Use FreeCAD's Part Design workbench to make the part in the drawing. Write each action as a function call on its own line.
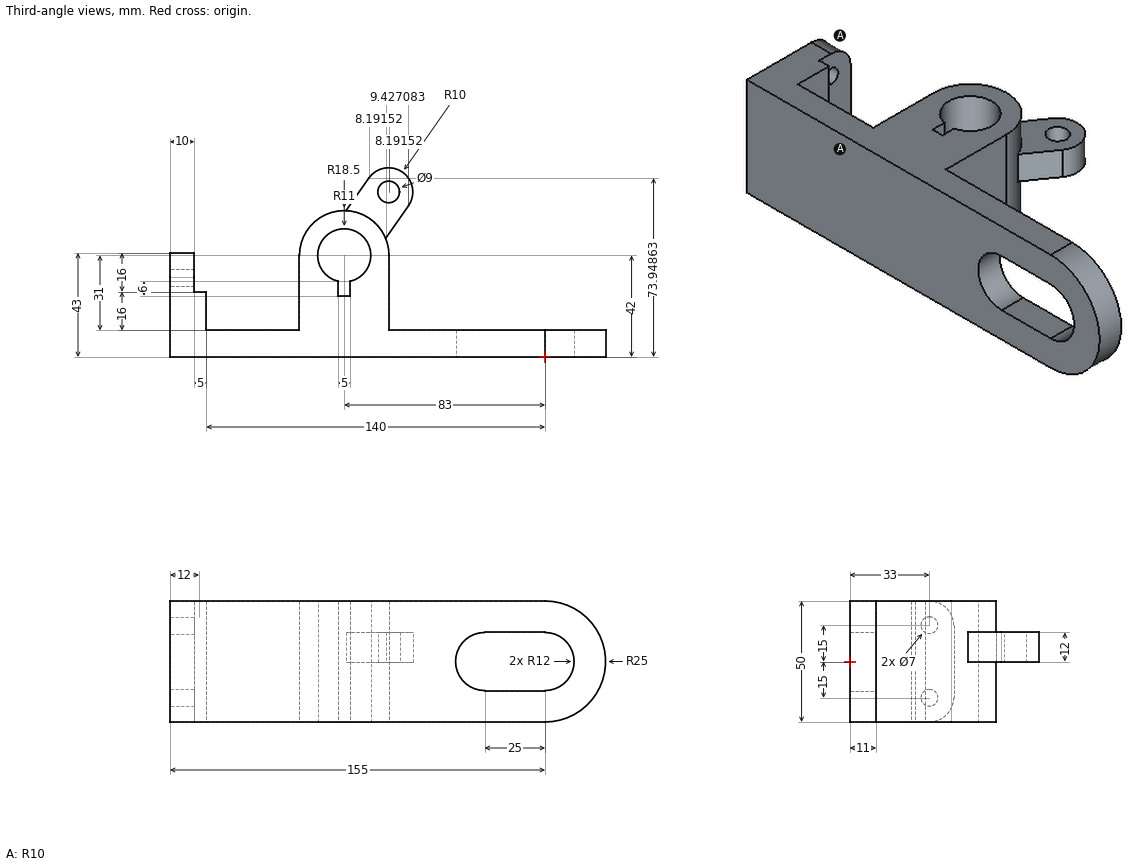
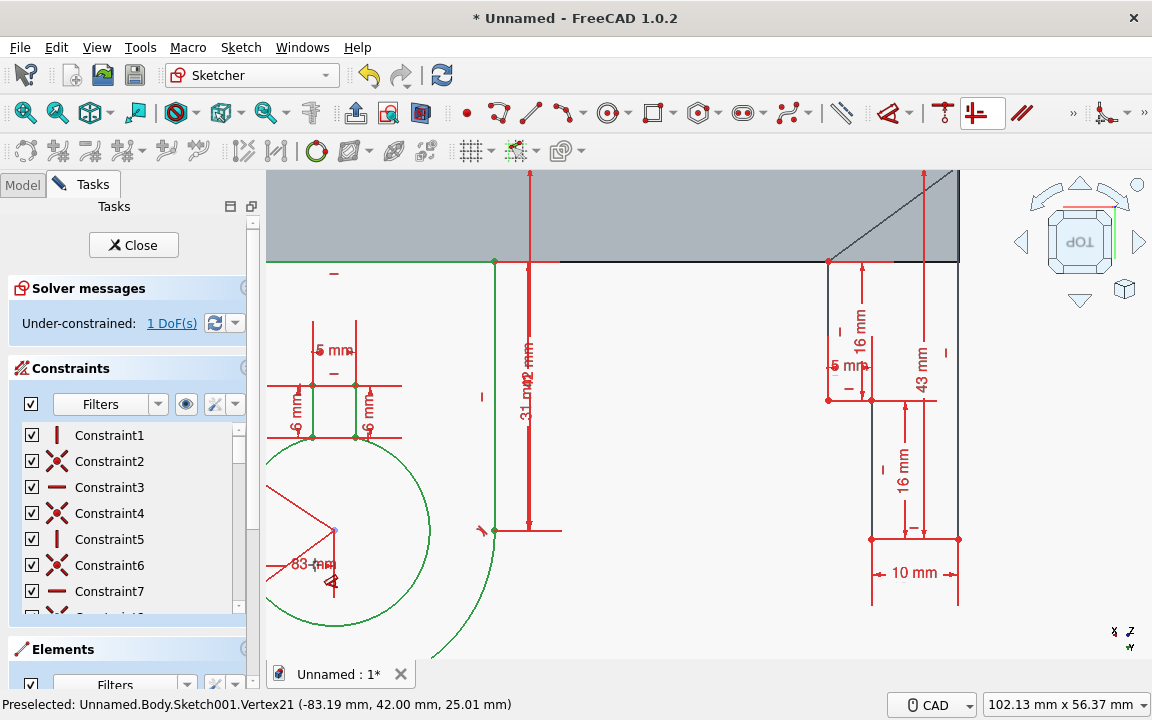
click(828, 262)
click(561, 296)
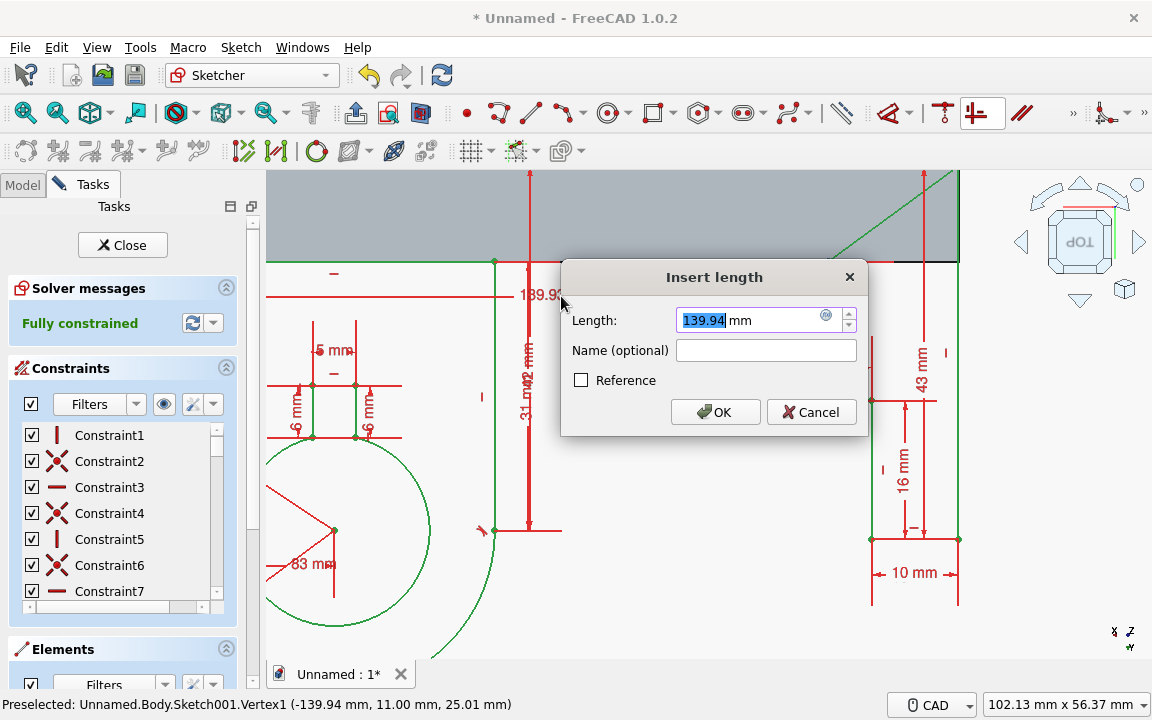
text(140)
key(Return)
key(Escape)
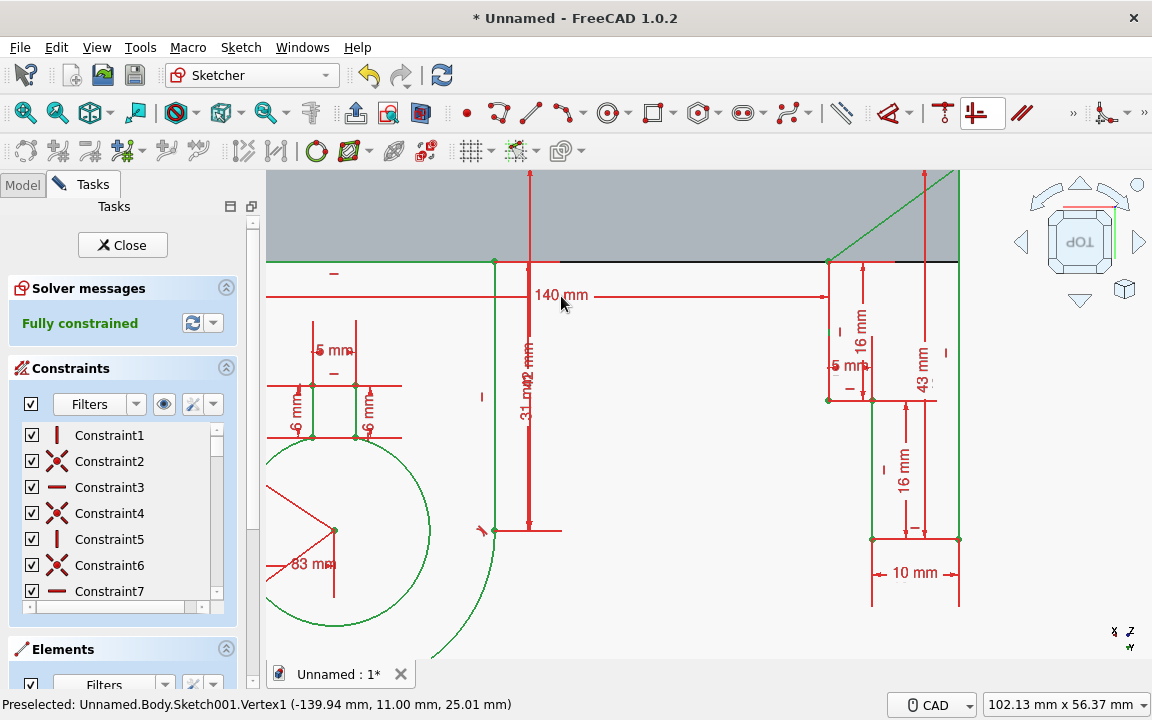
click(123, 245)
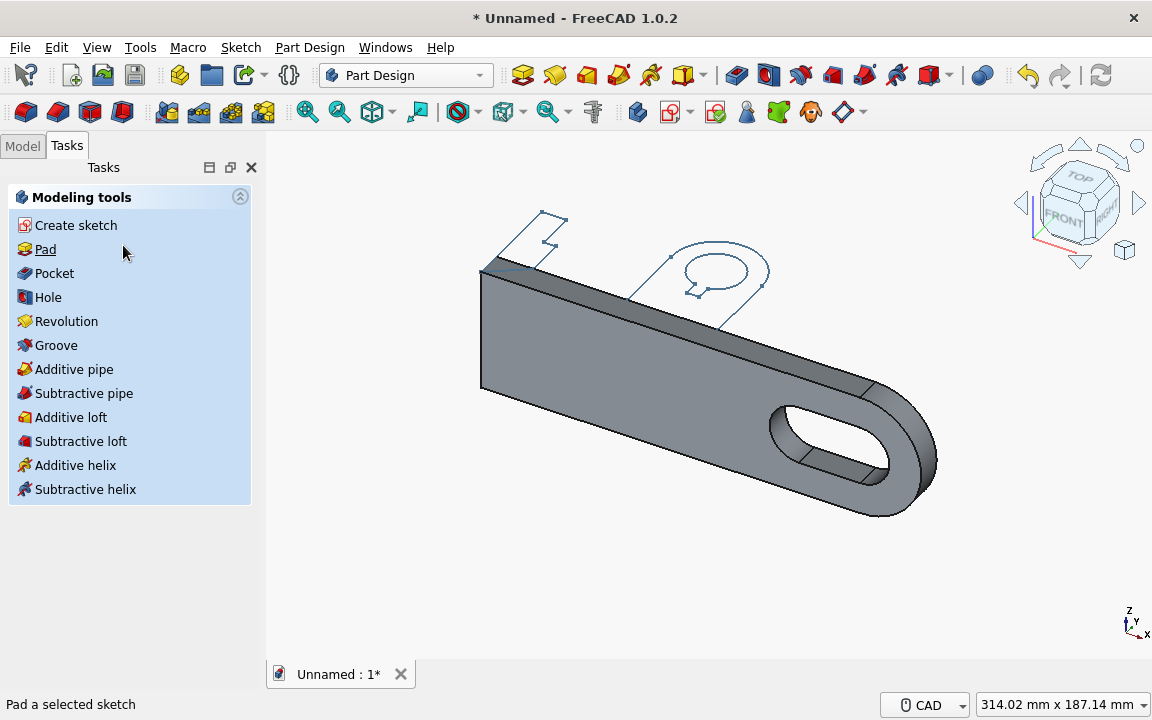
click(524, 76)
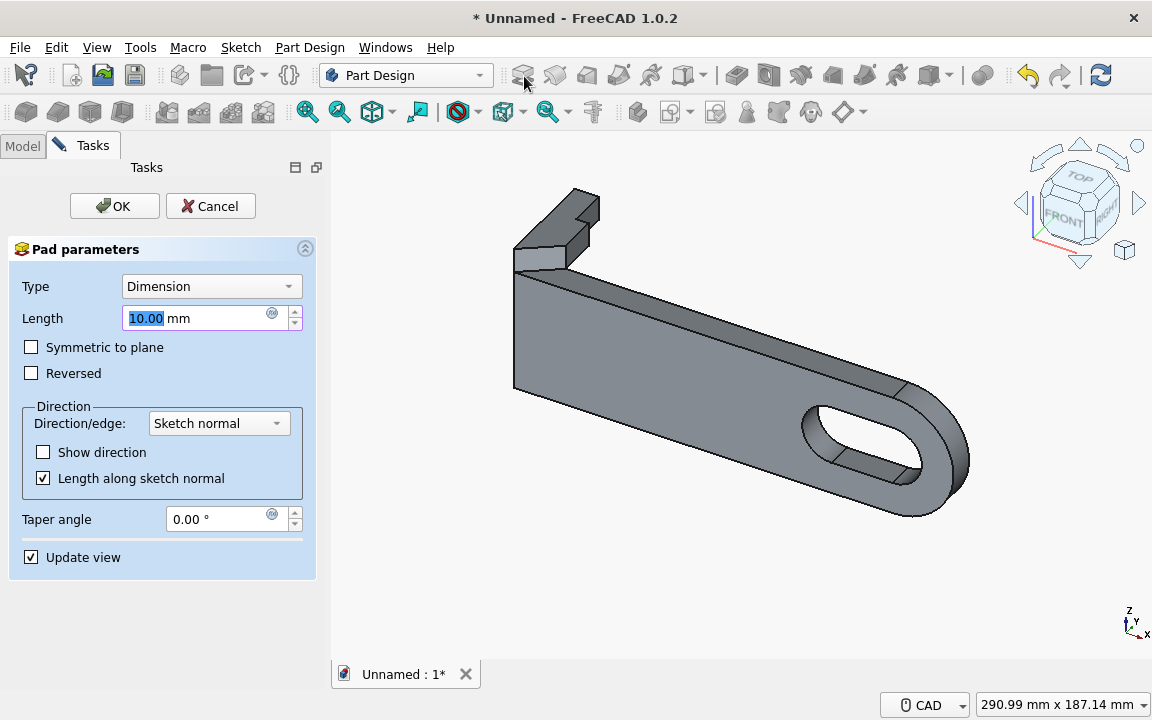
text(50)
key(Tab)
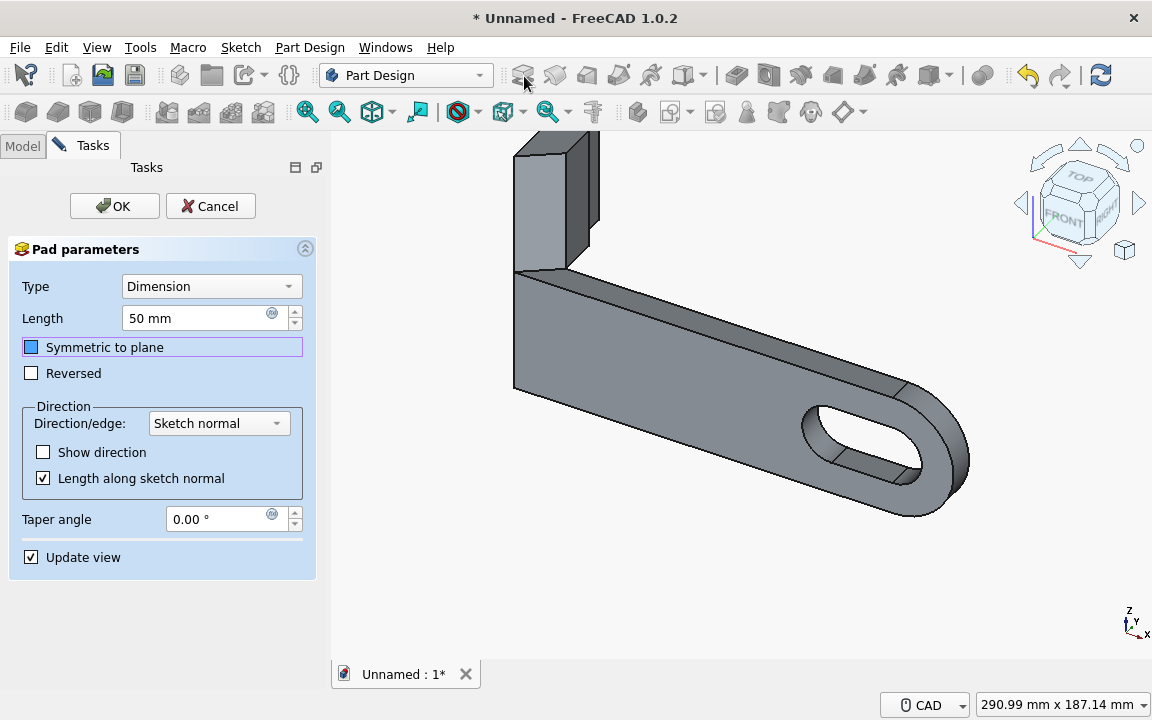
click(30, 373)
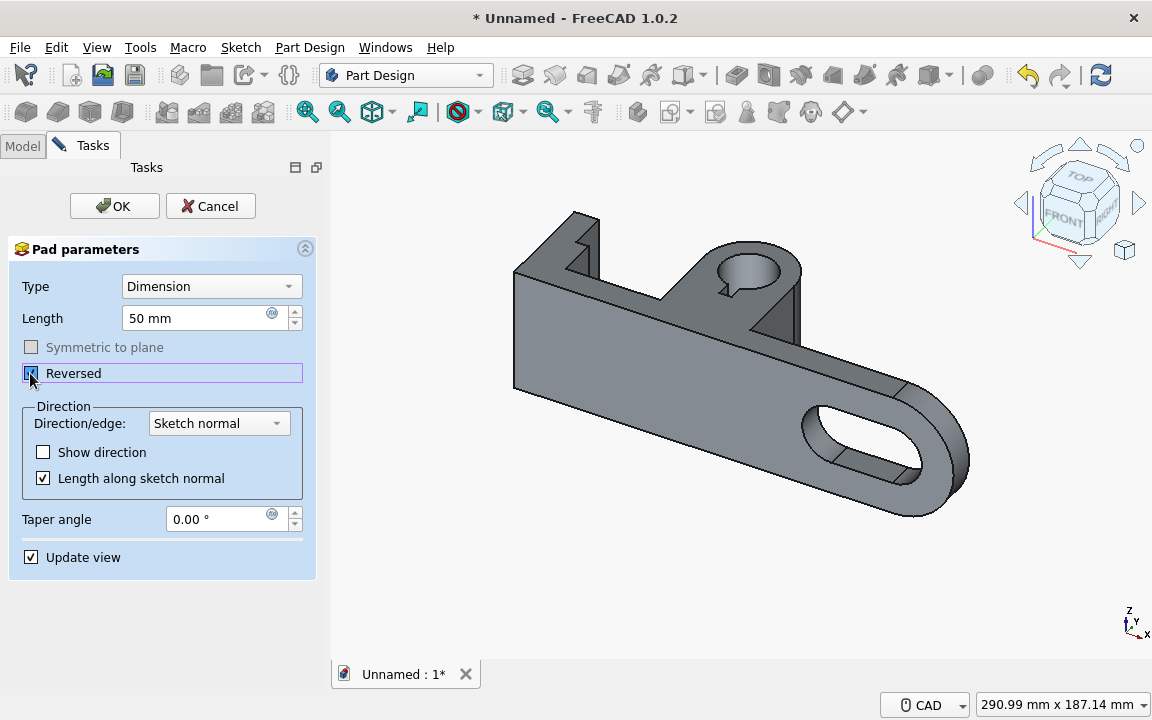
click(115, 206)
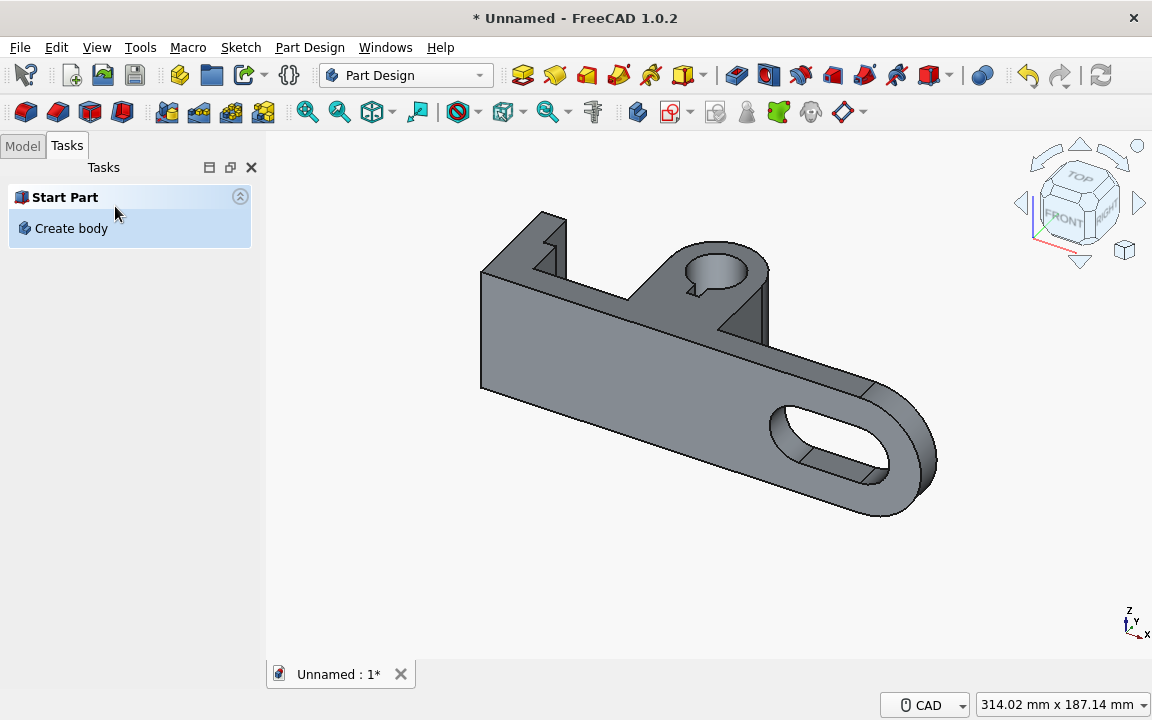
click(23, 145)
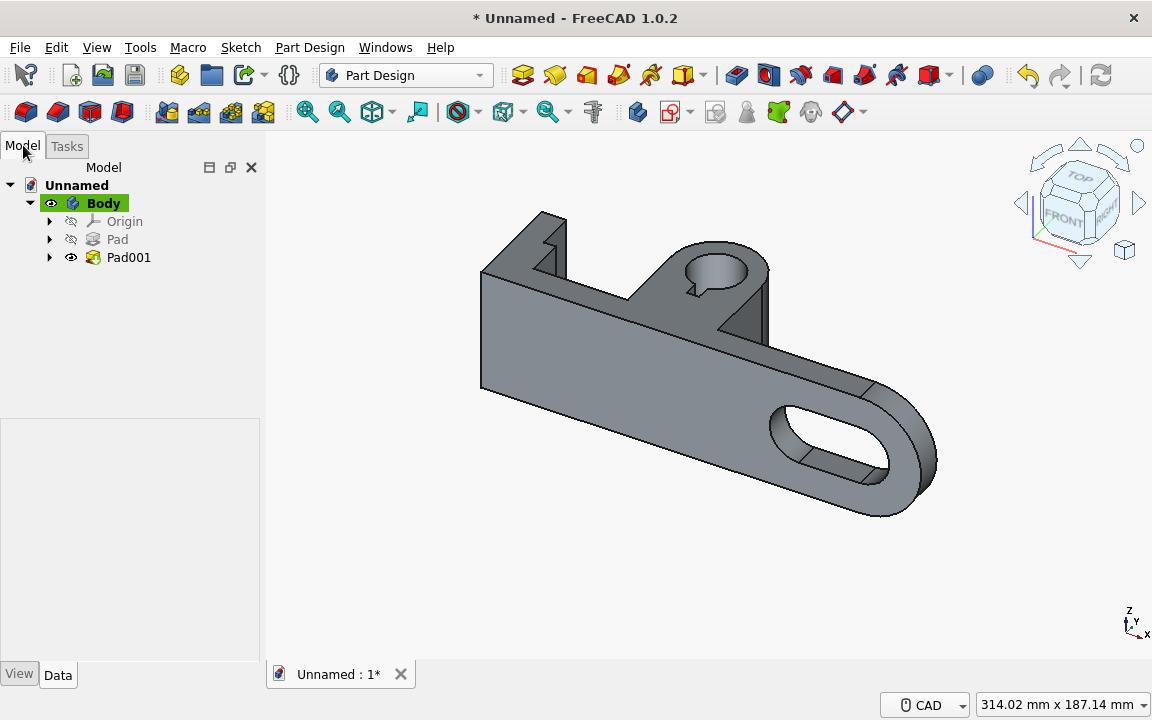
click(50, 221)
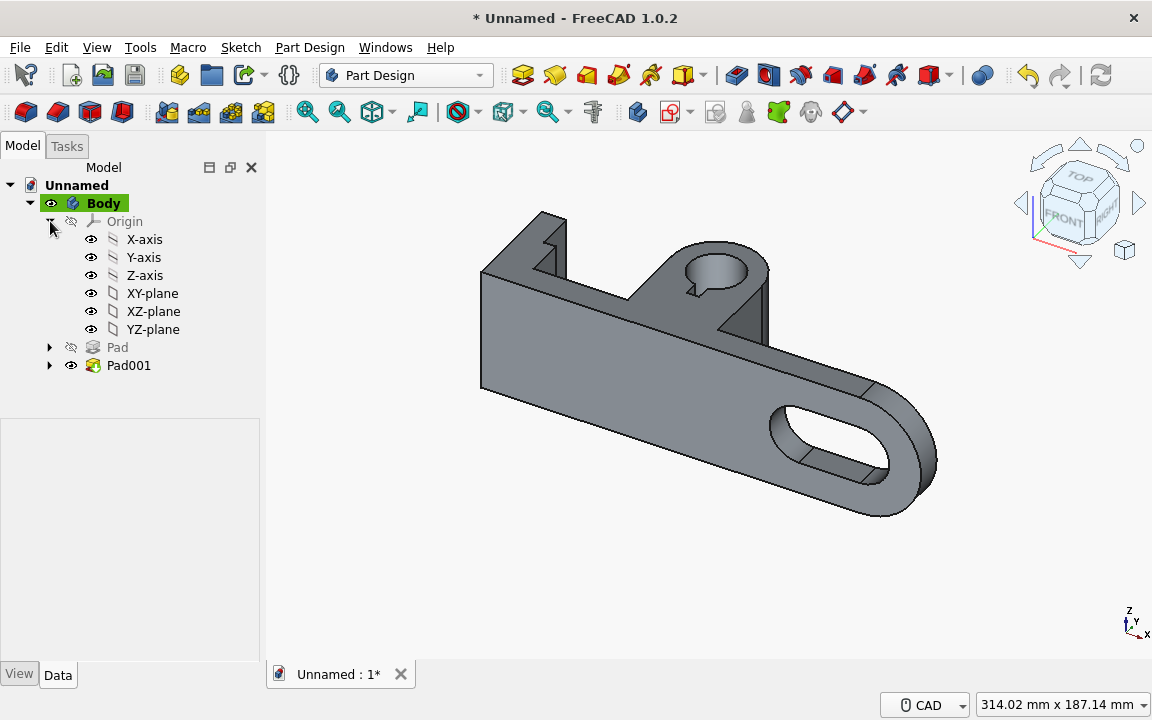
click(136, 293)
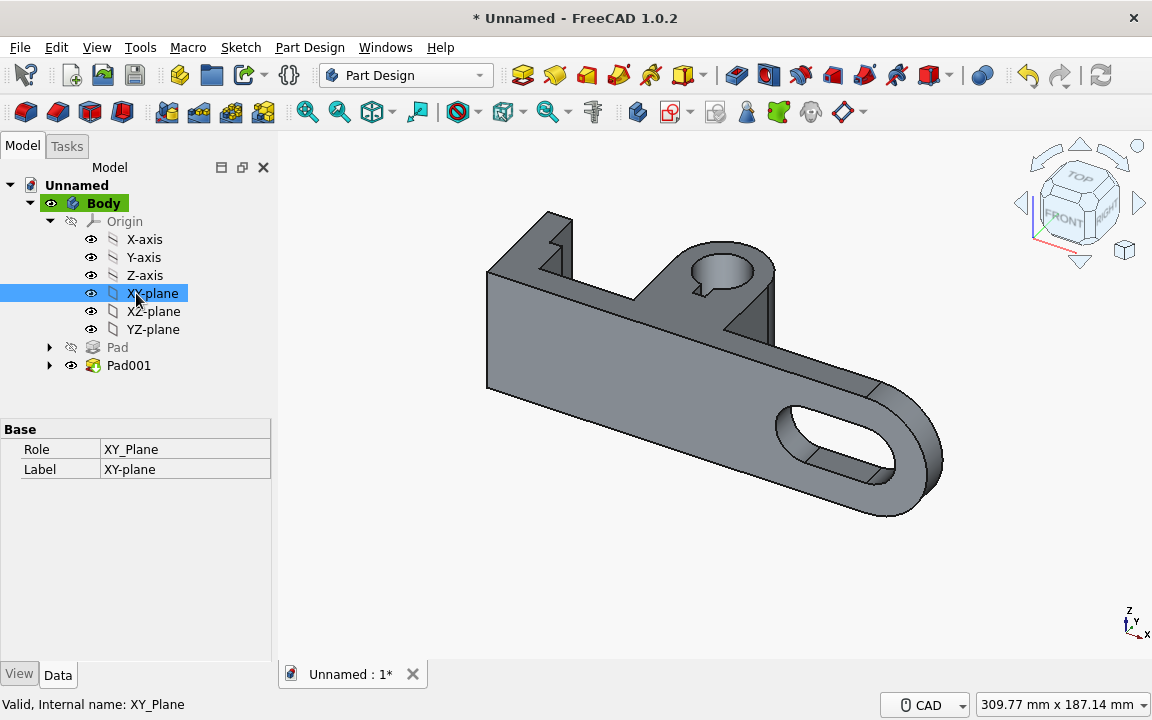
click(844, 112)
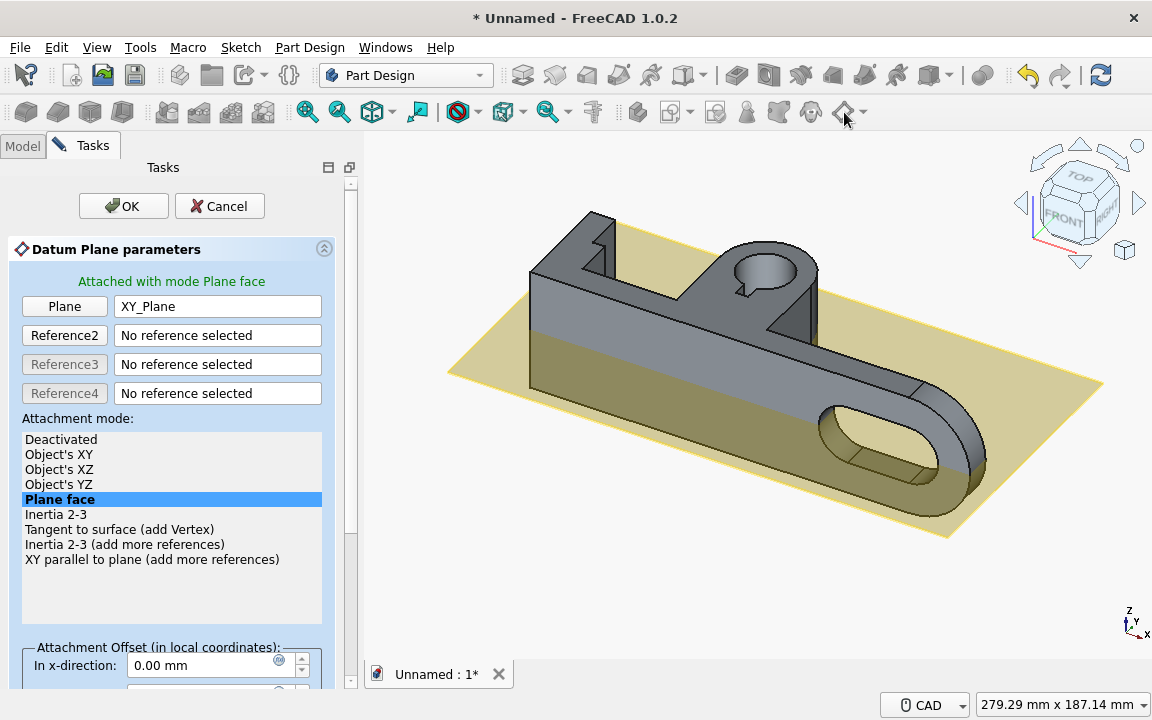
scroll(351, 432, down, 2)